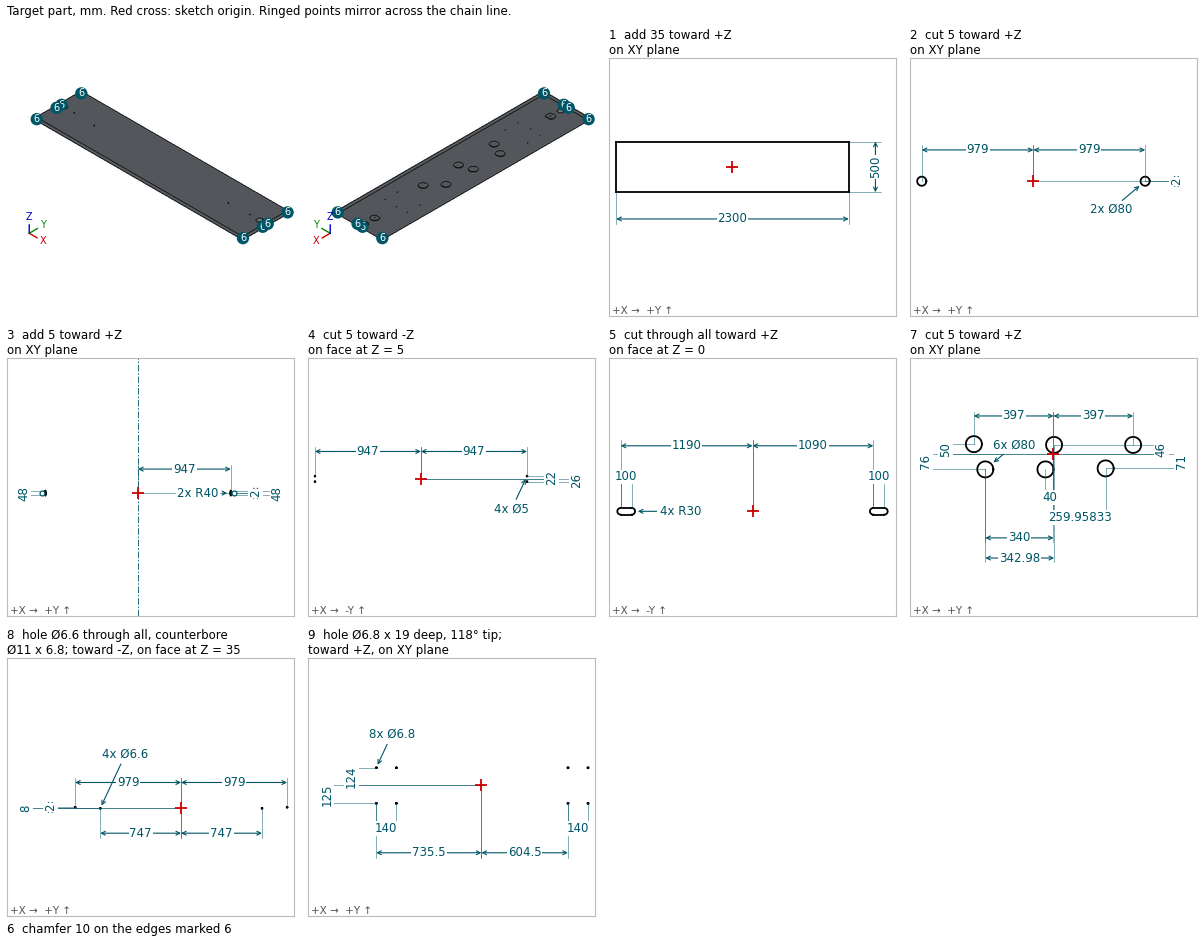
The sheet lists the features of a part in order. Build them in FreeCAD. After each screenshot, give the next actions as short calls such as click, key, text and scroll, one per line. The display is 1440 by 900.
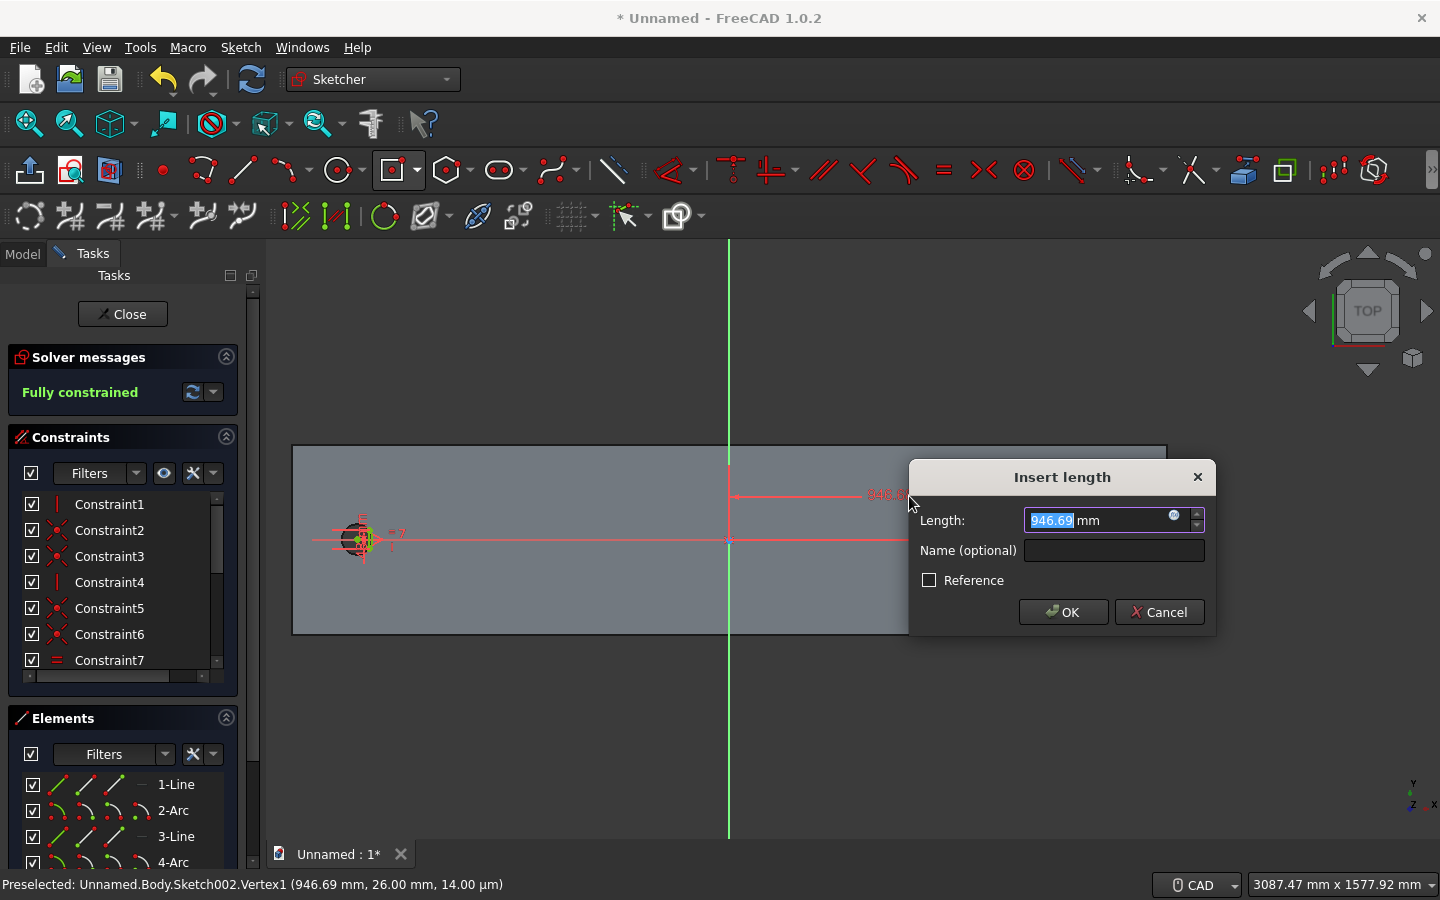
text(947)
key(Return)
key(Escape)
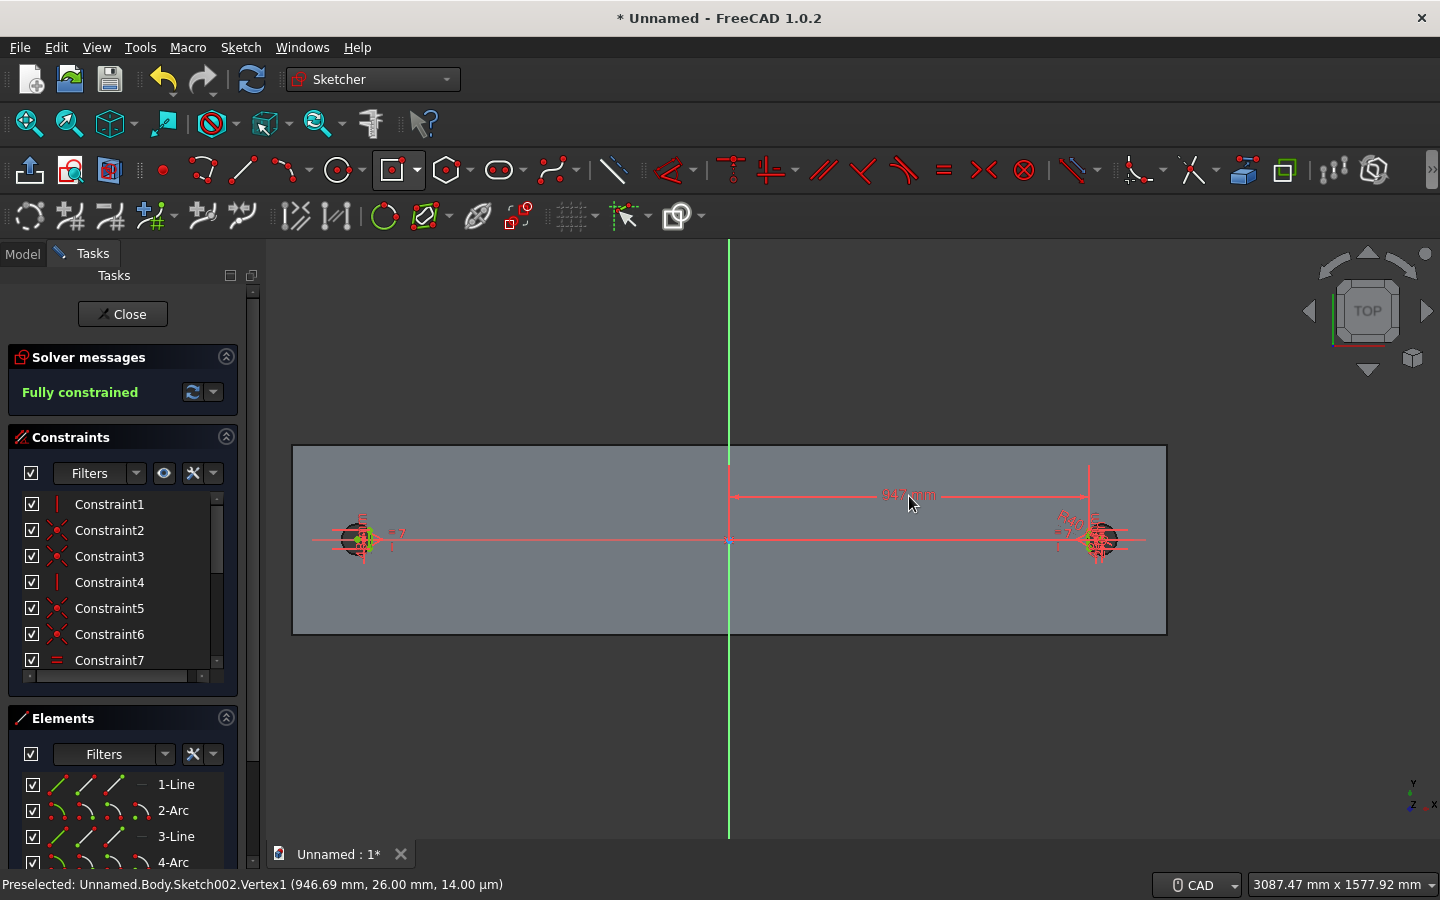
click(123, 314)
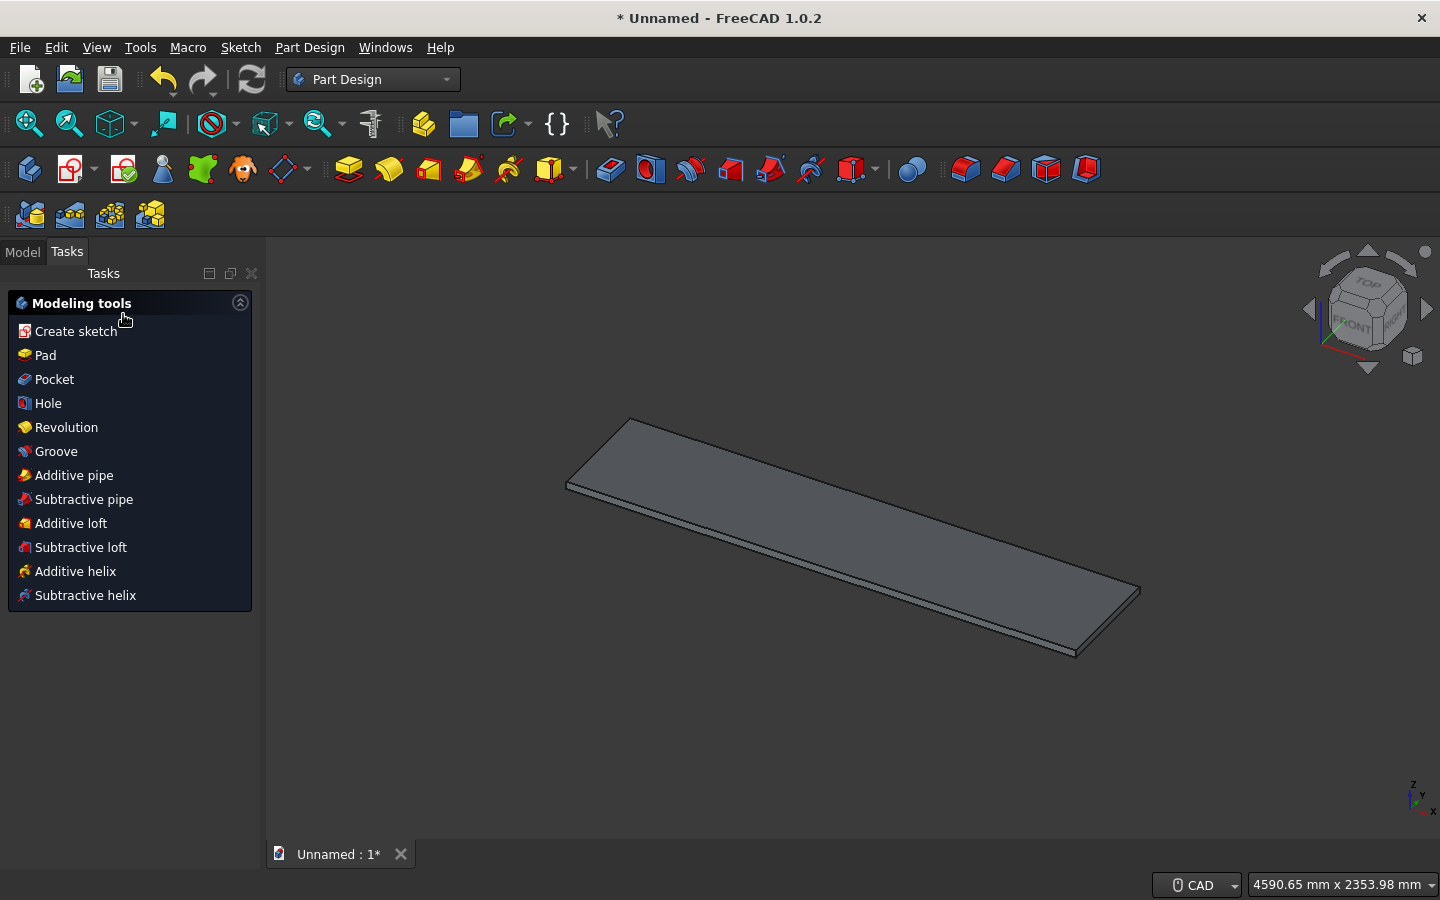
click(350, 170)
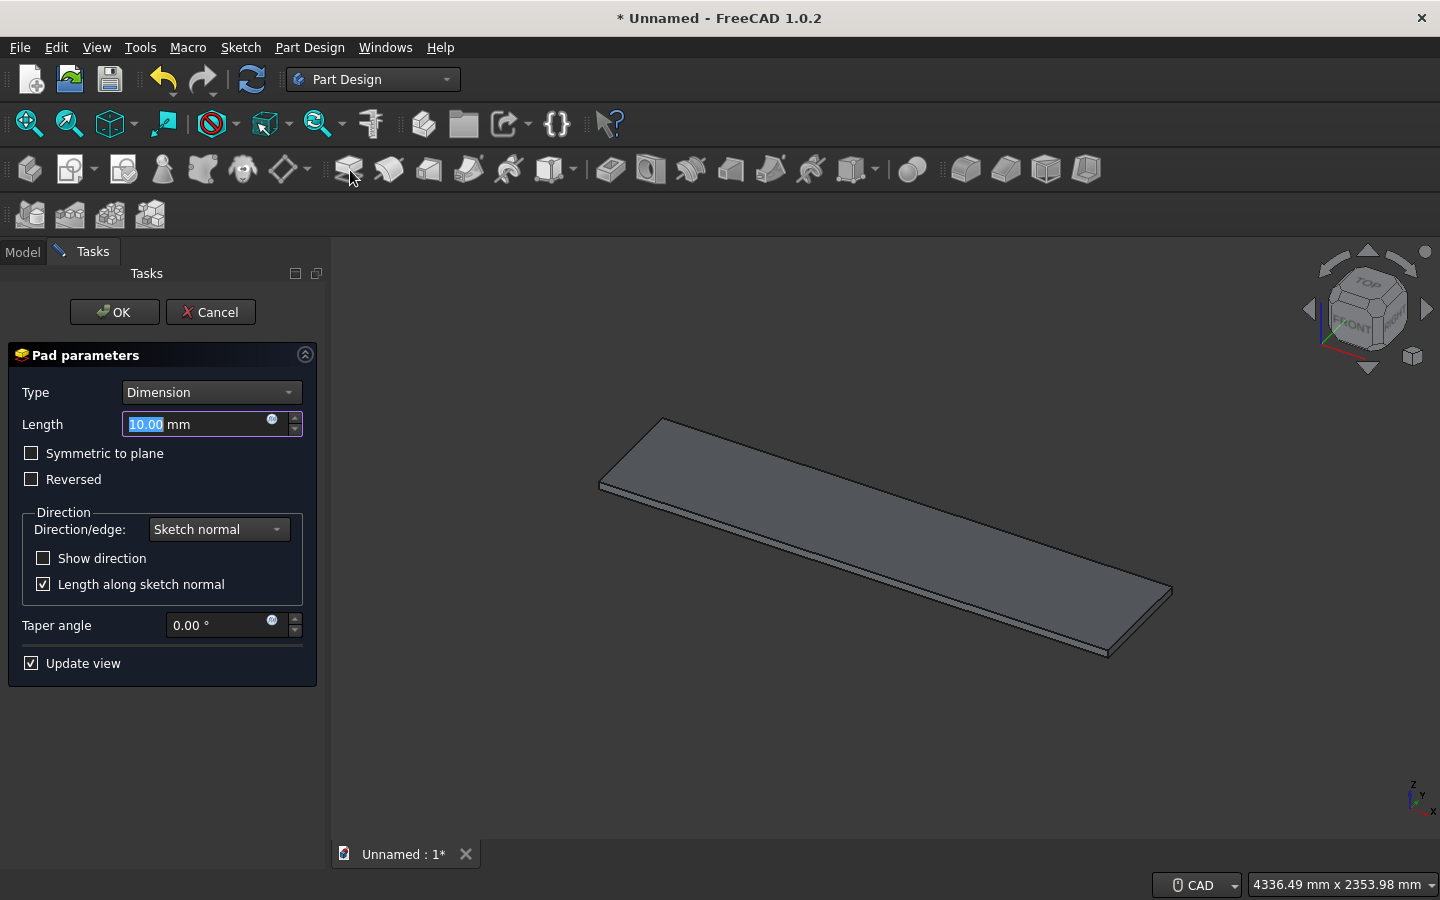
text(5)
key(Tab)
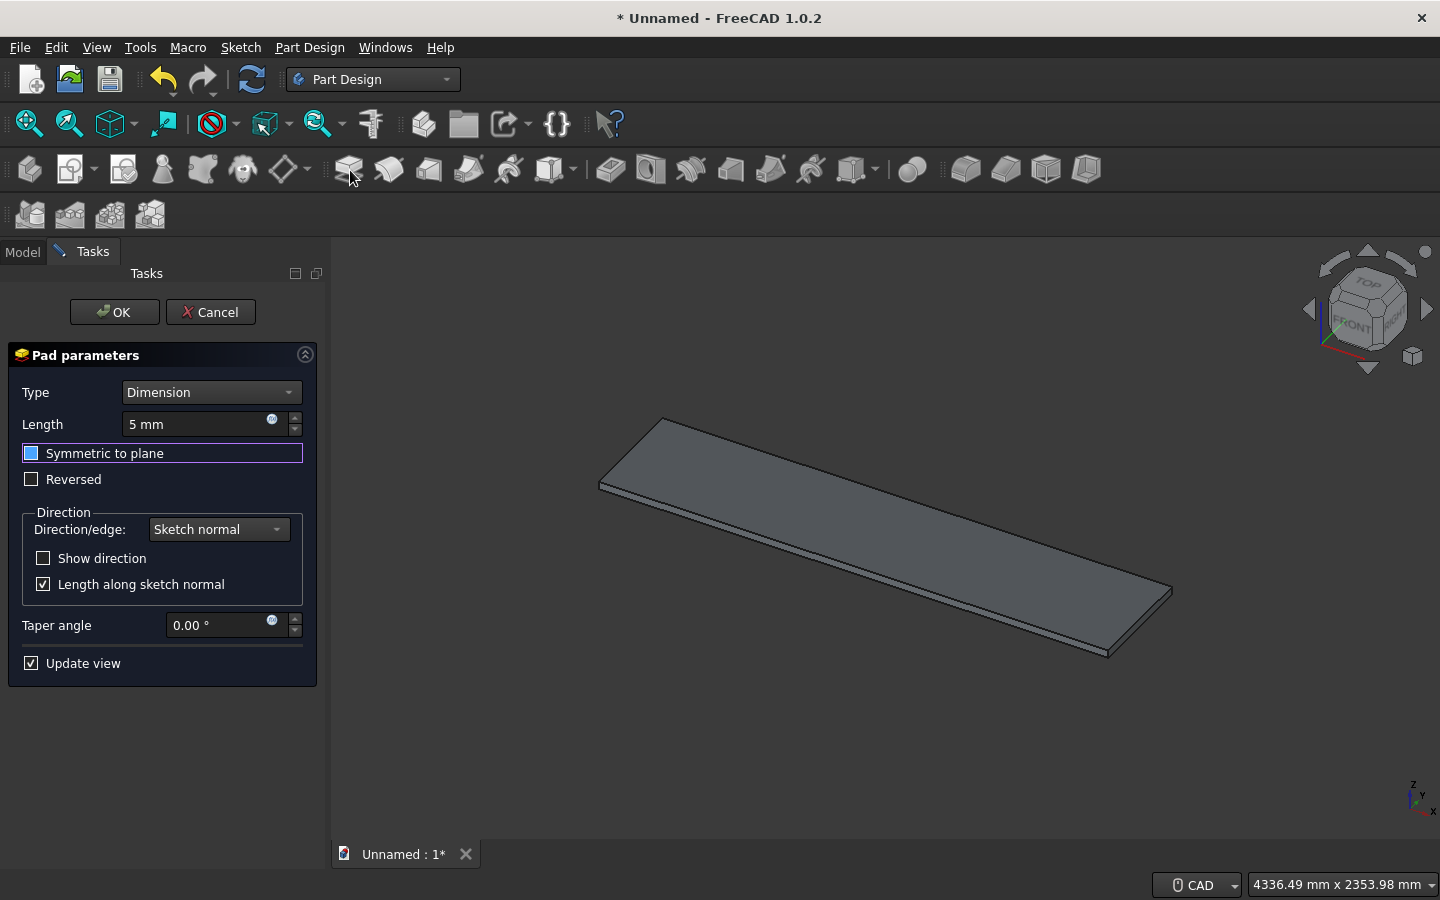
click(115, 312)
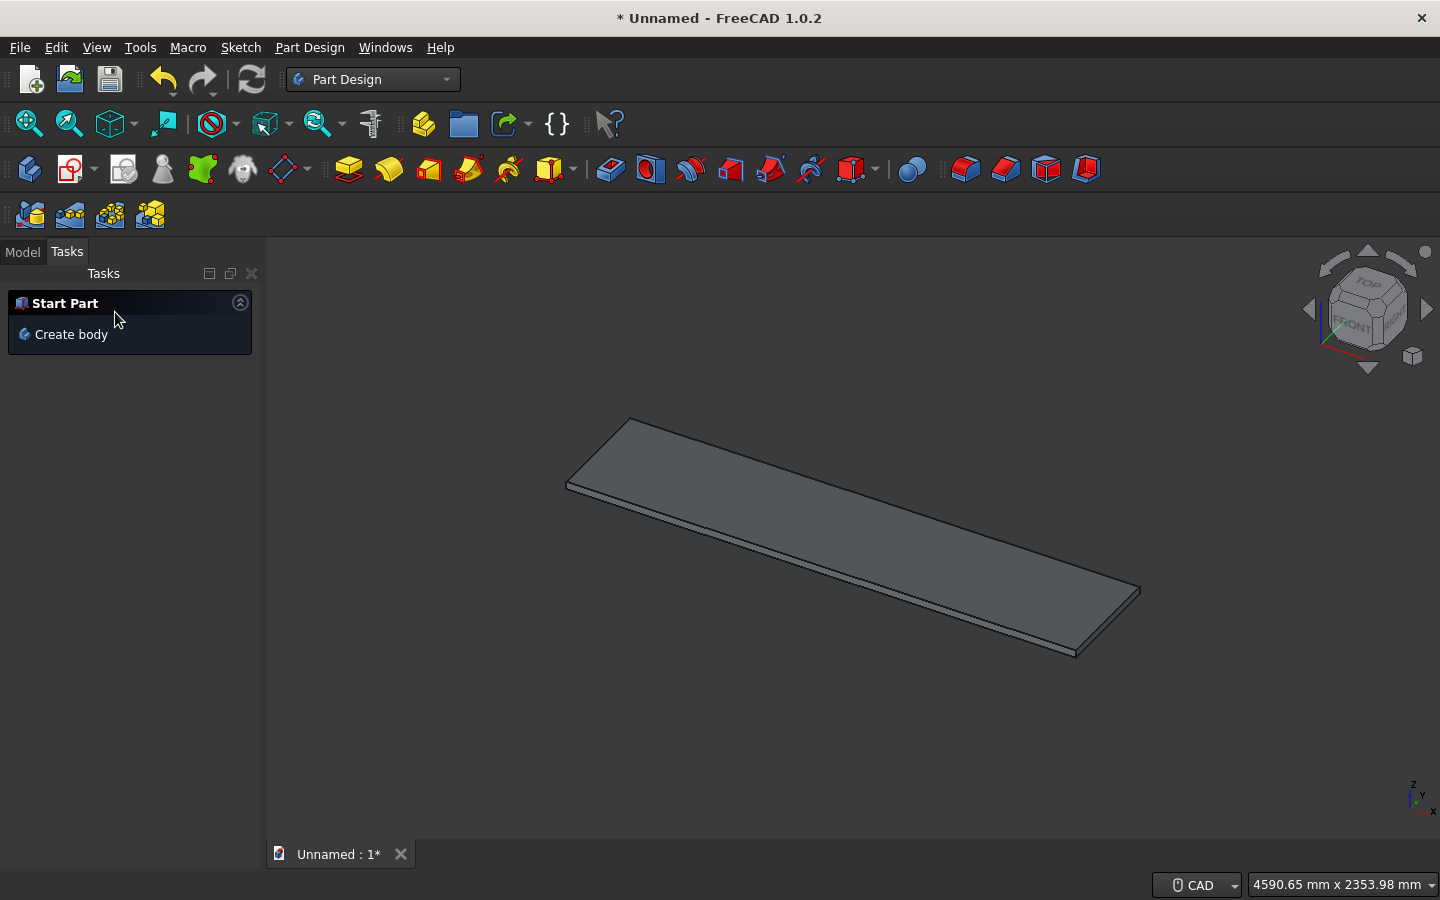
key(5)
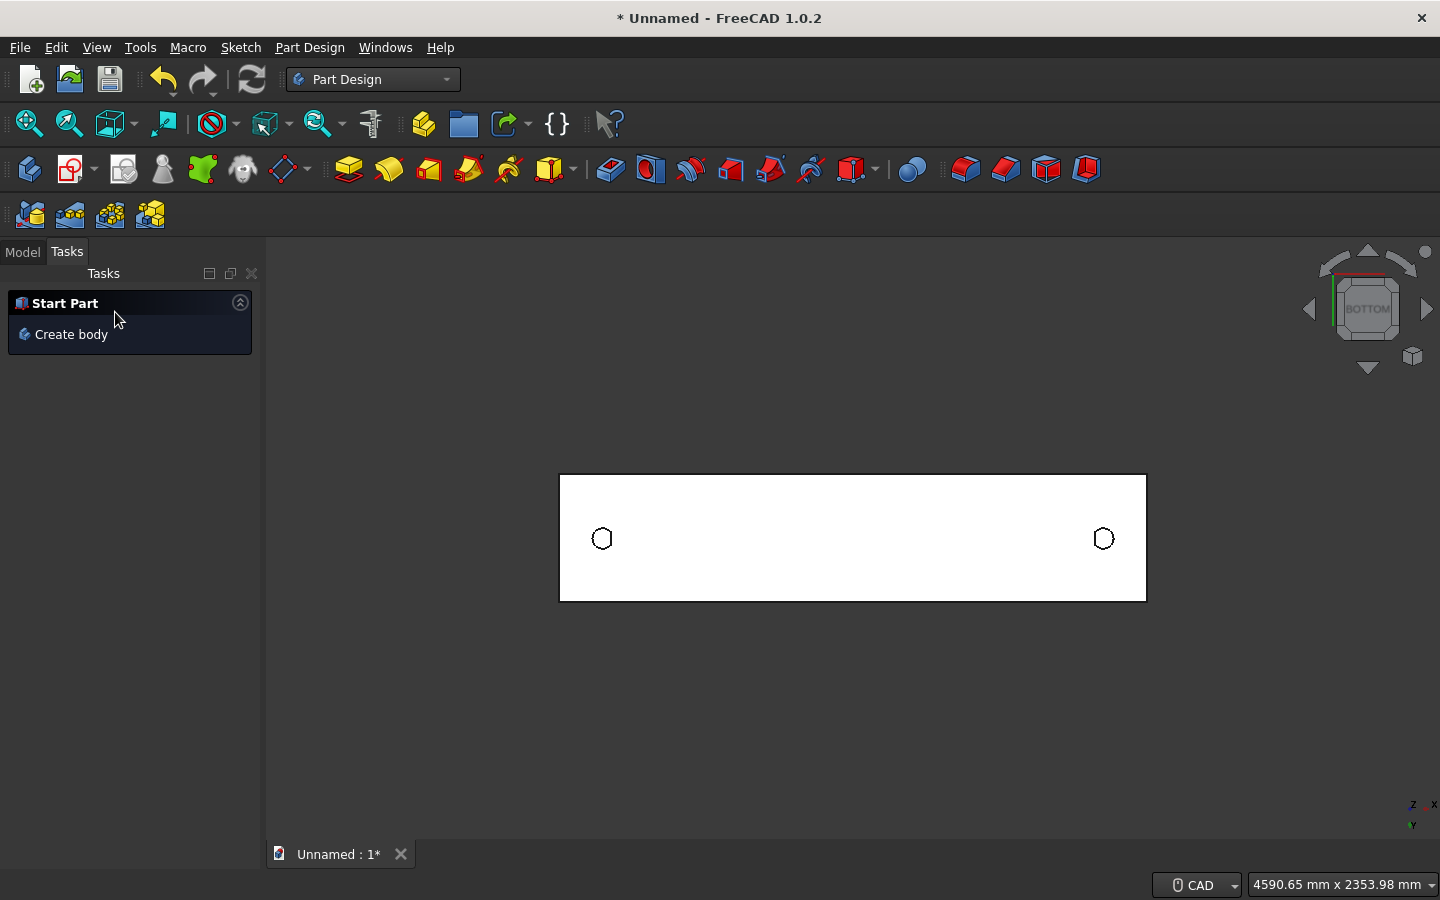
click(1104, 538)